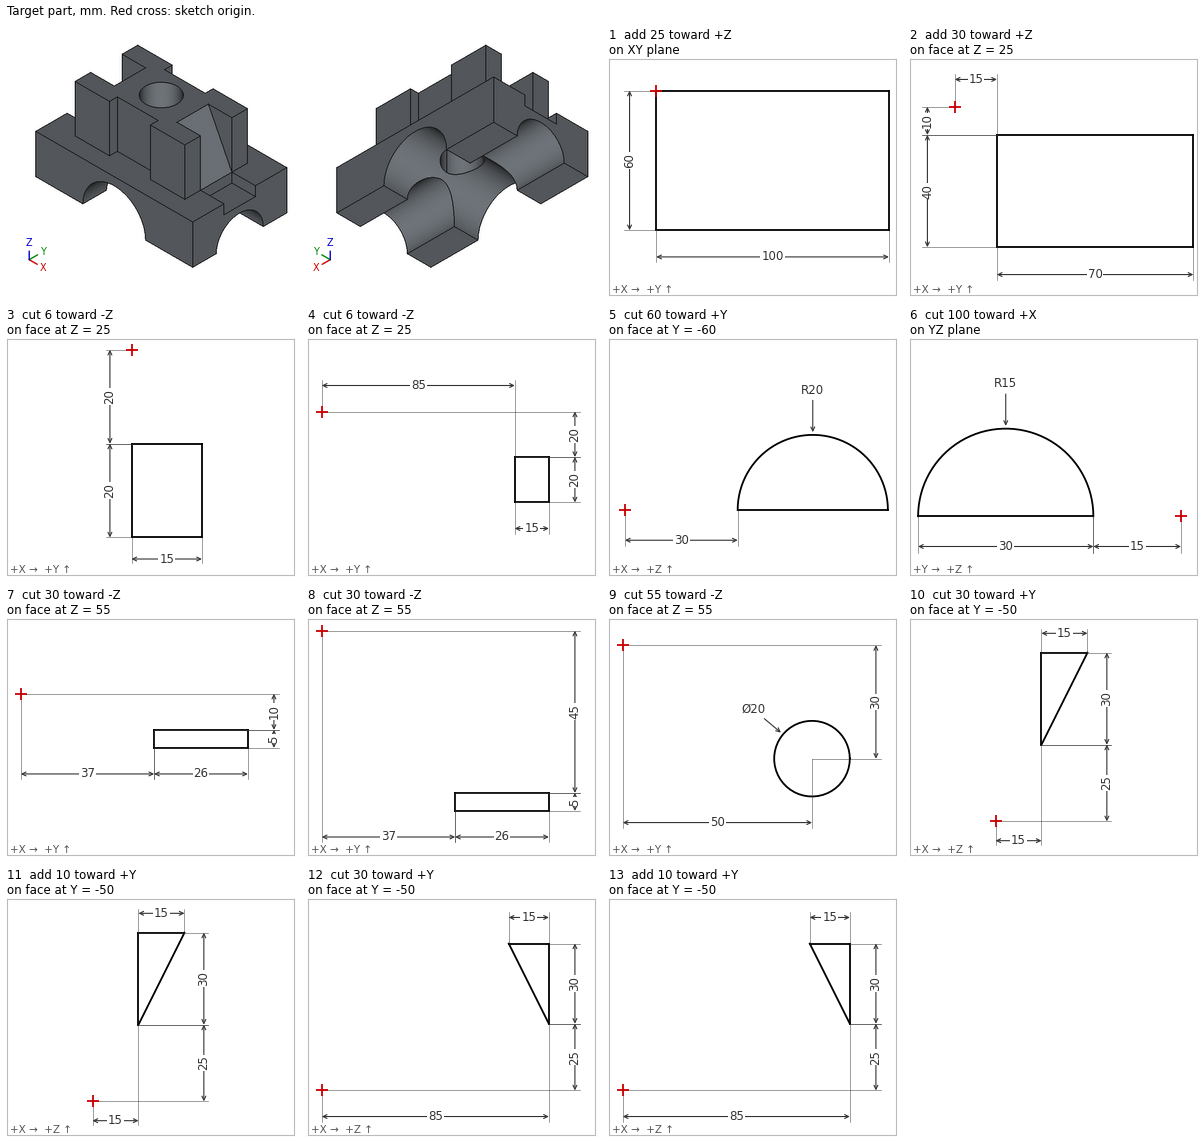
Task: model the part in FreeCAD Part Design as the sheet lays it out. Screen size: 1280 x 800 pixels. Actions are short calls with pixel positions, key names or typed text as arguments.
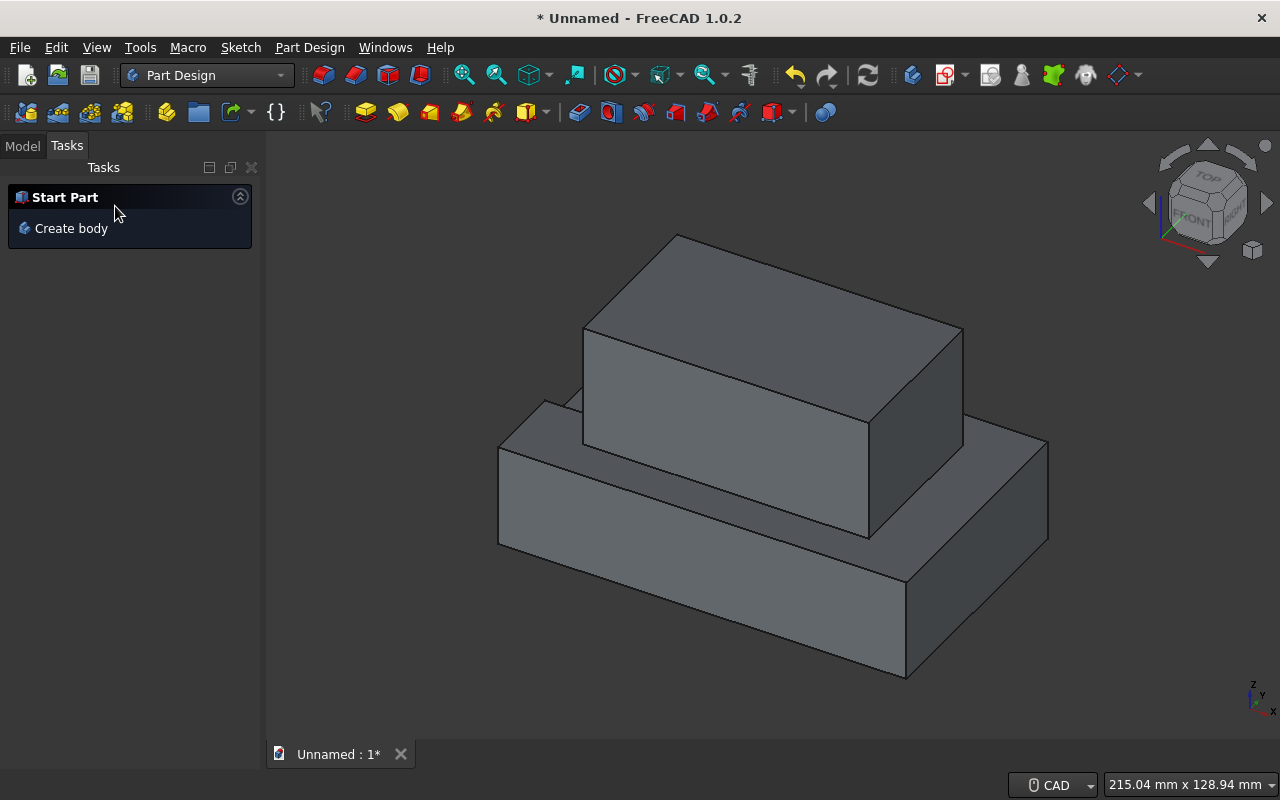
click(988, 461)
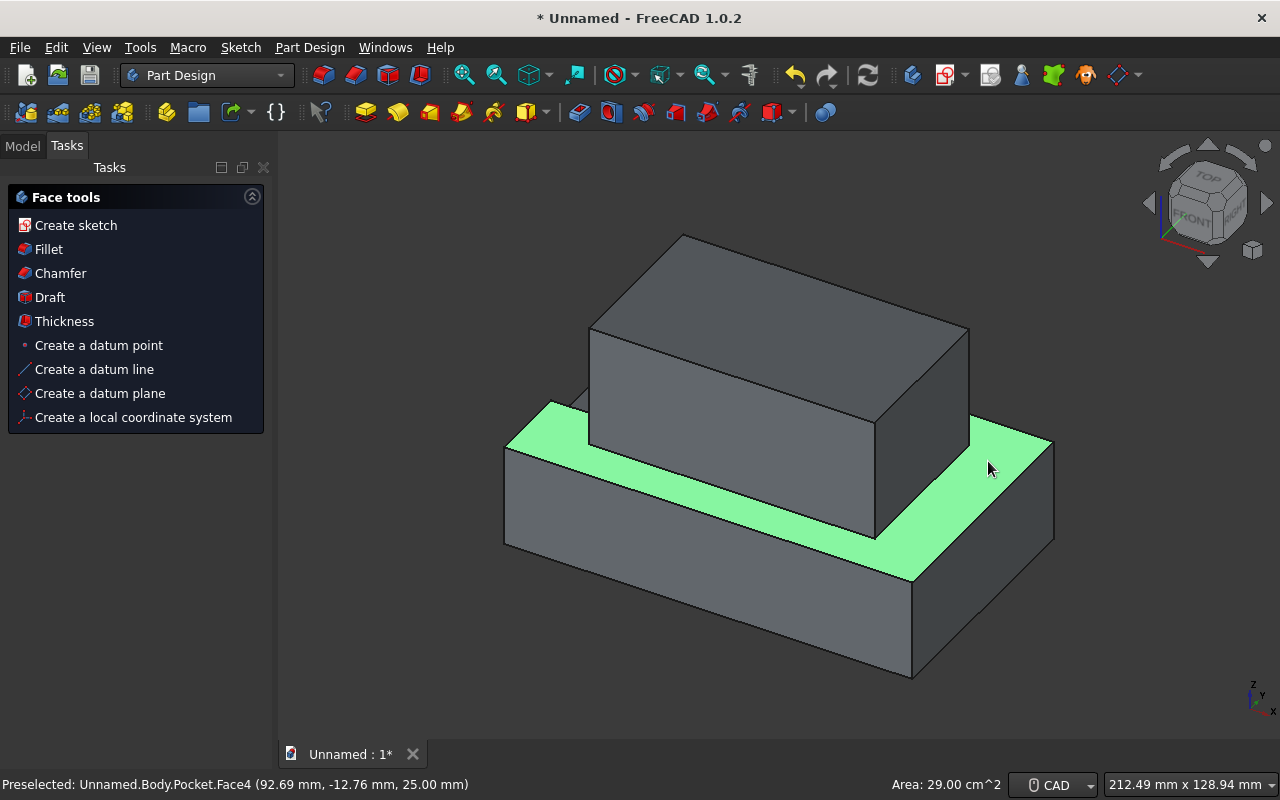
click(946, 76)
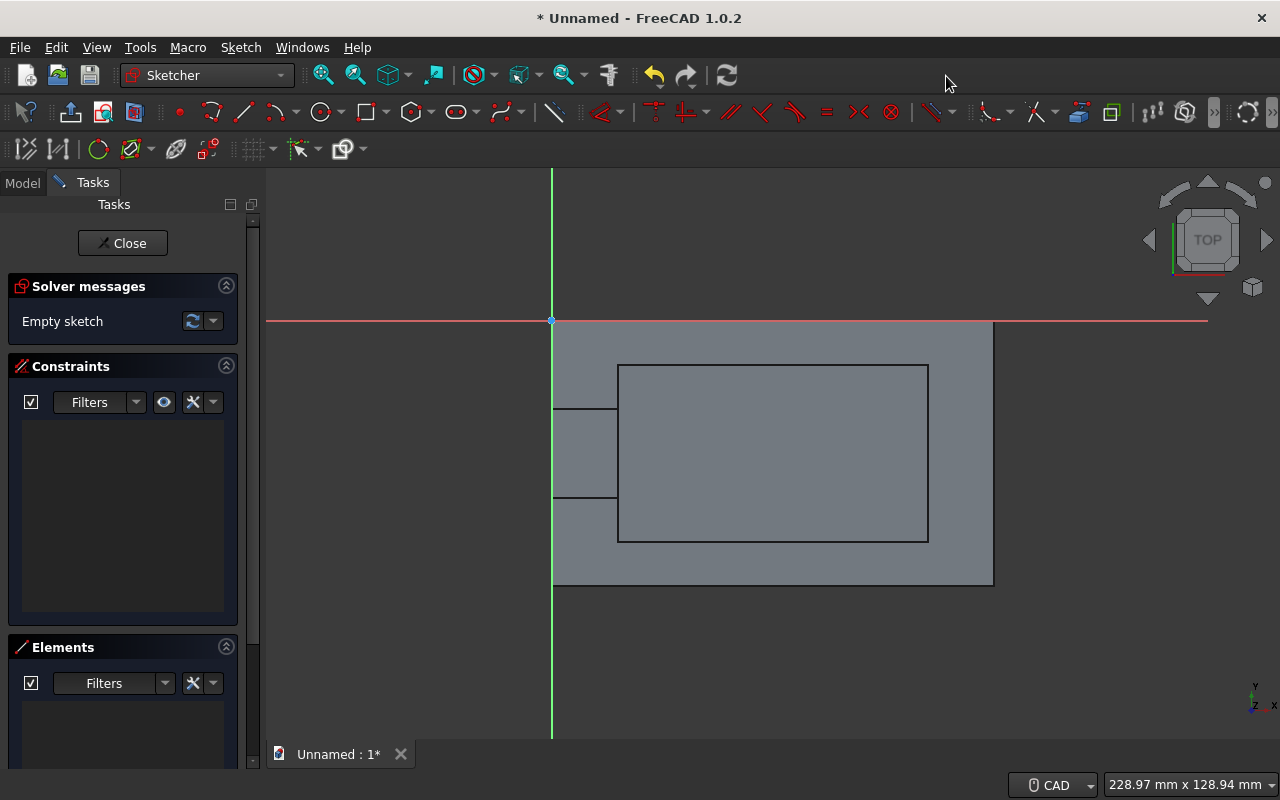
scroll(1045, 454, up, 7)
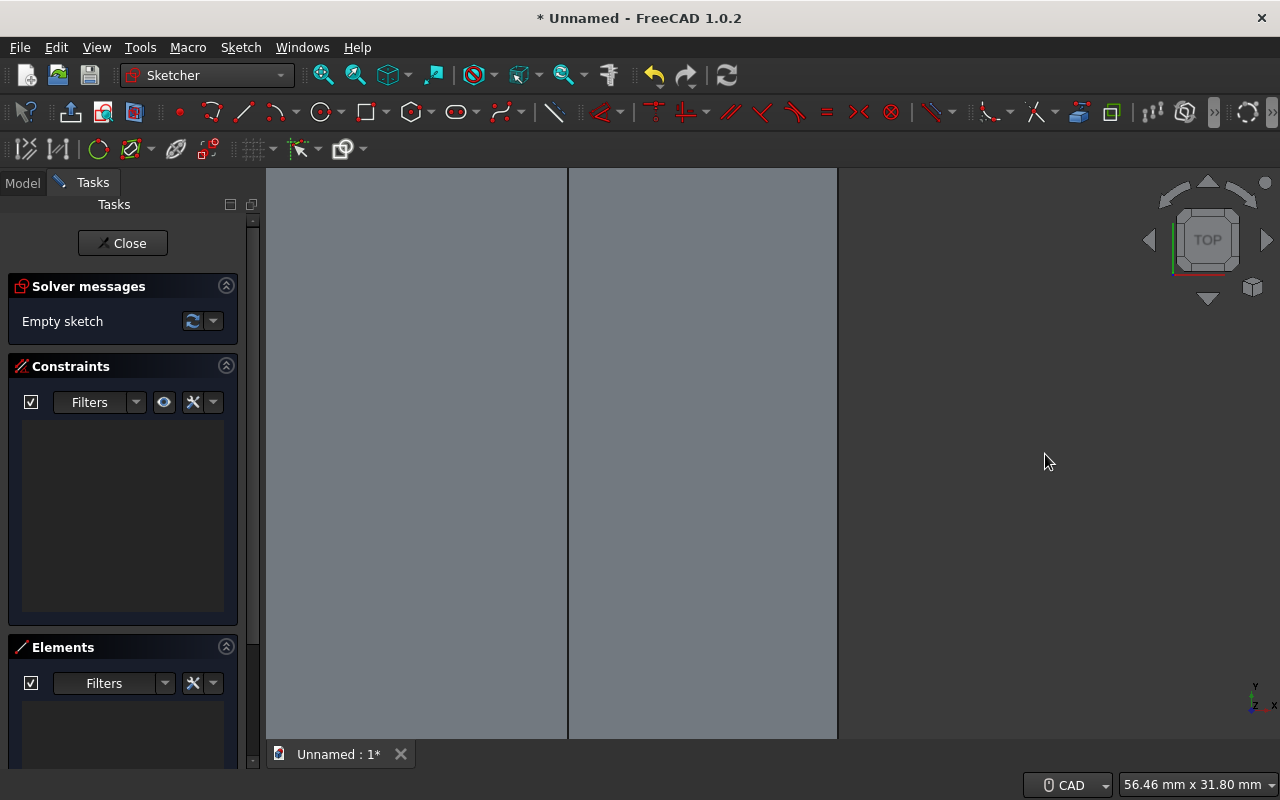
key(g)
key(r)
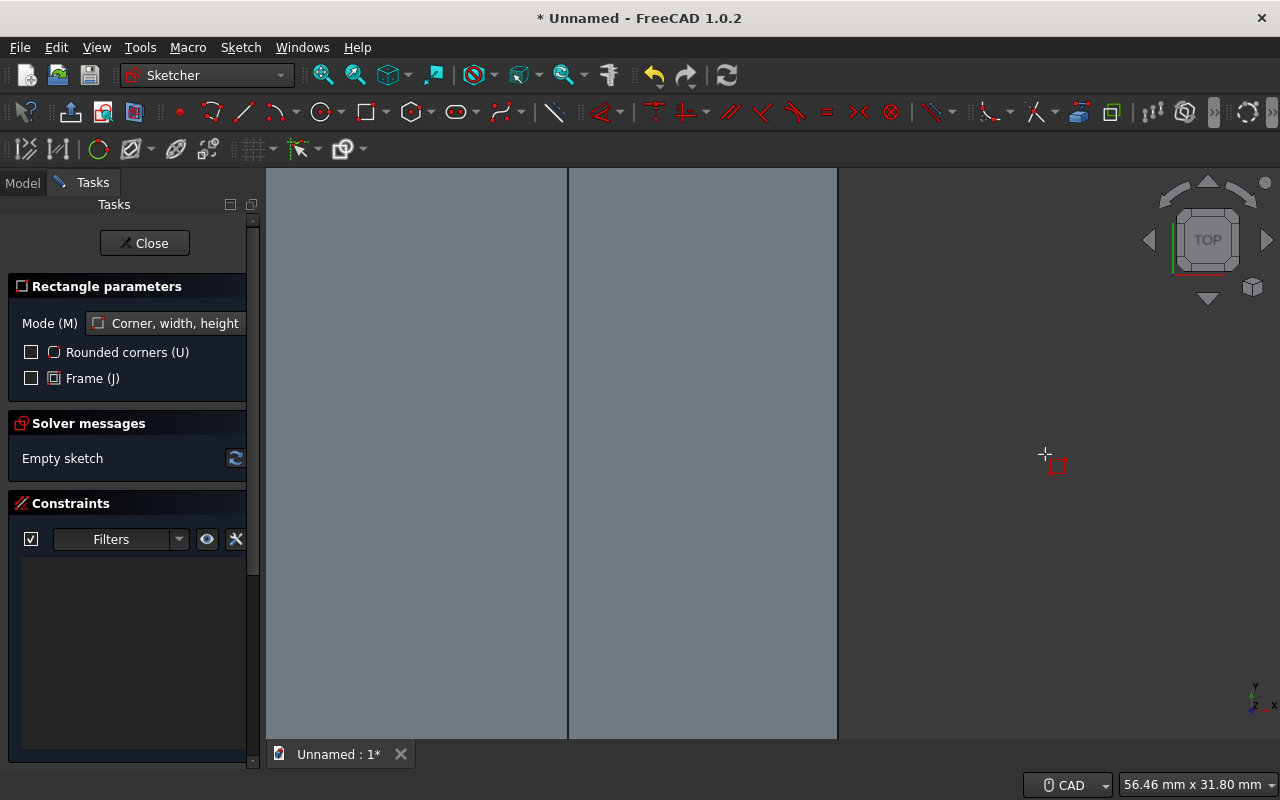
click(568, 271)
click(838, 630)
key(Escape)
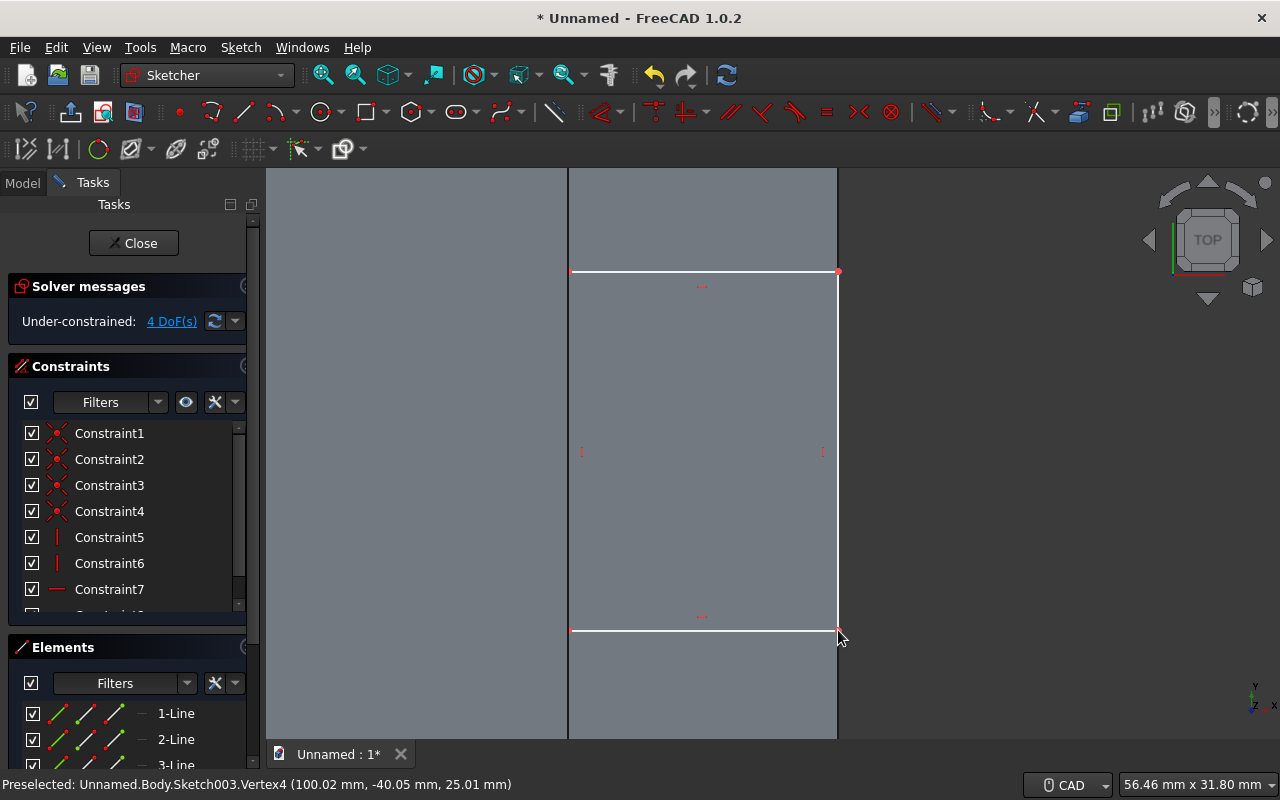
click(600, 112)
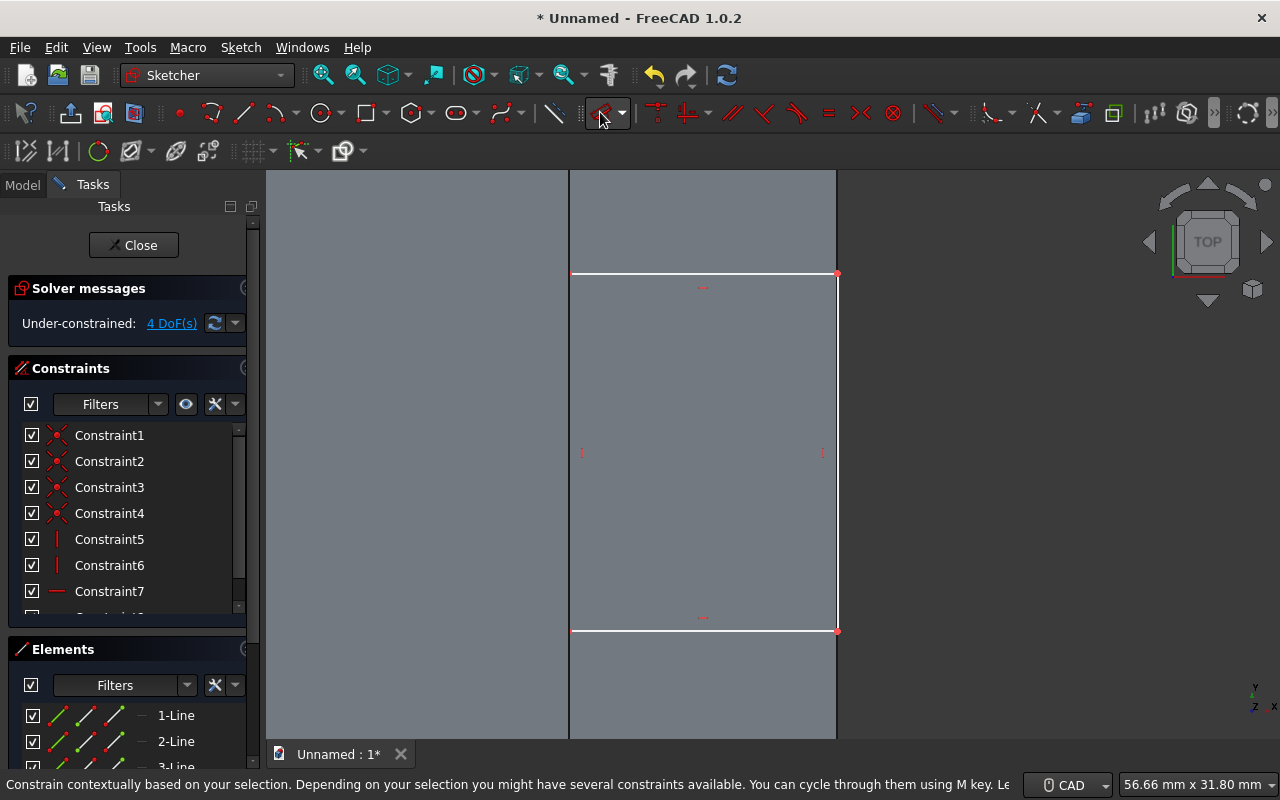
click(569, 381)
click(535, 453)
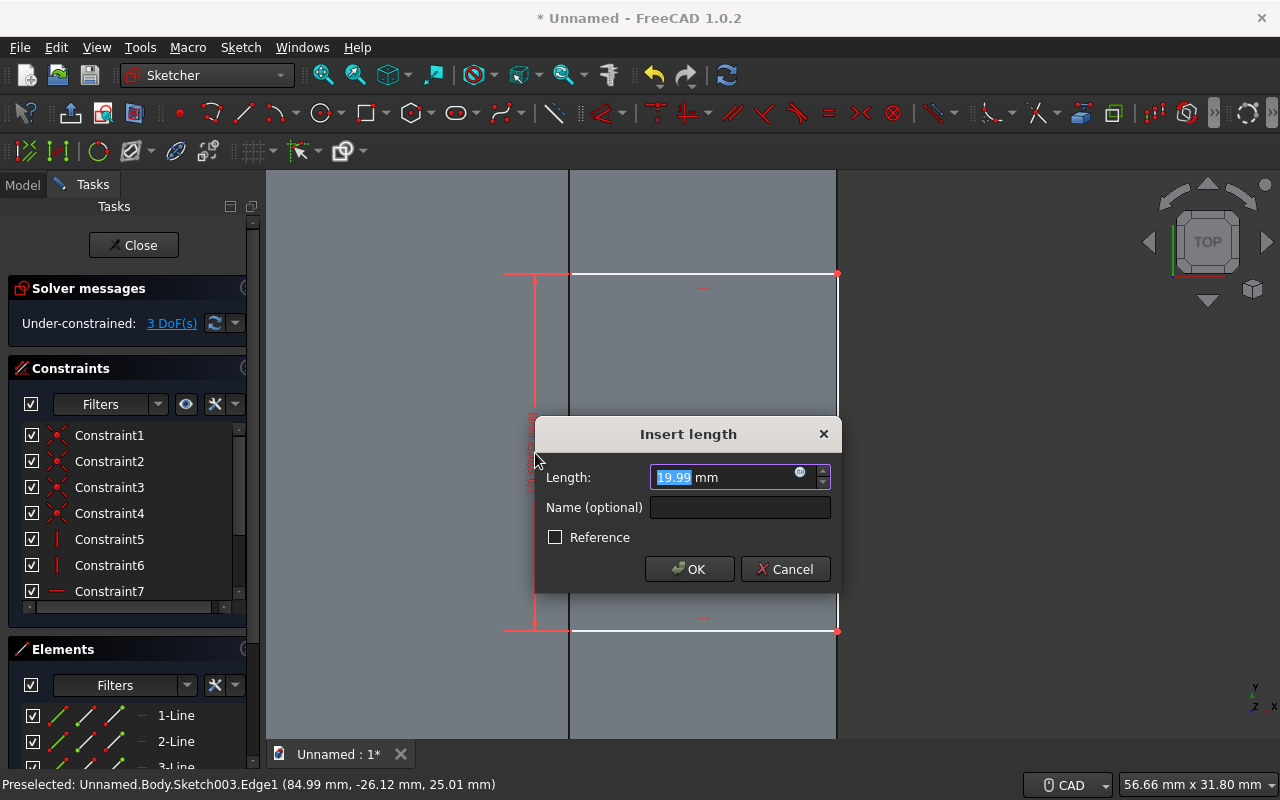
text(20)
key(Return)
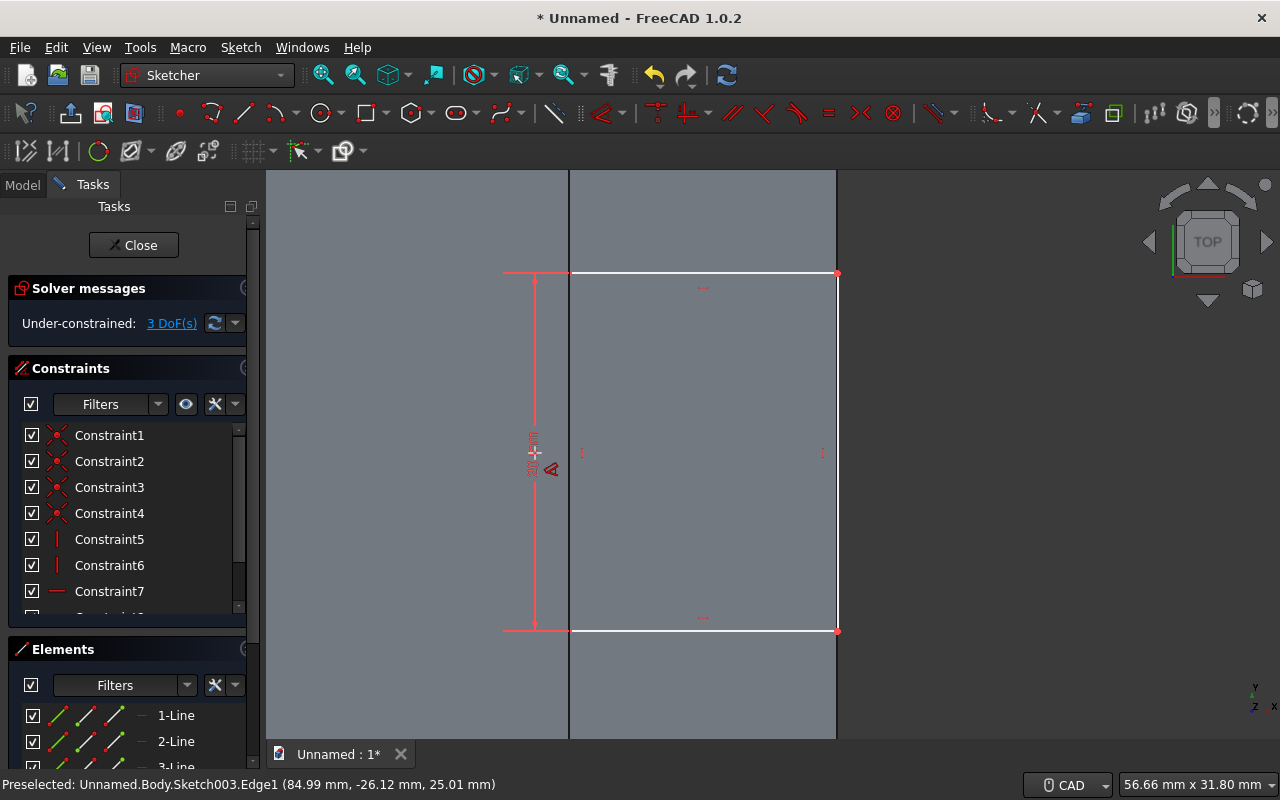
click(649, 631)
click(703, 665)